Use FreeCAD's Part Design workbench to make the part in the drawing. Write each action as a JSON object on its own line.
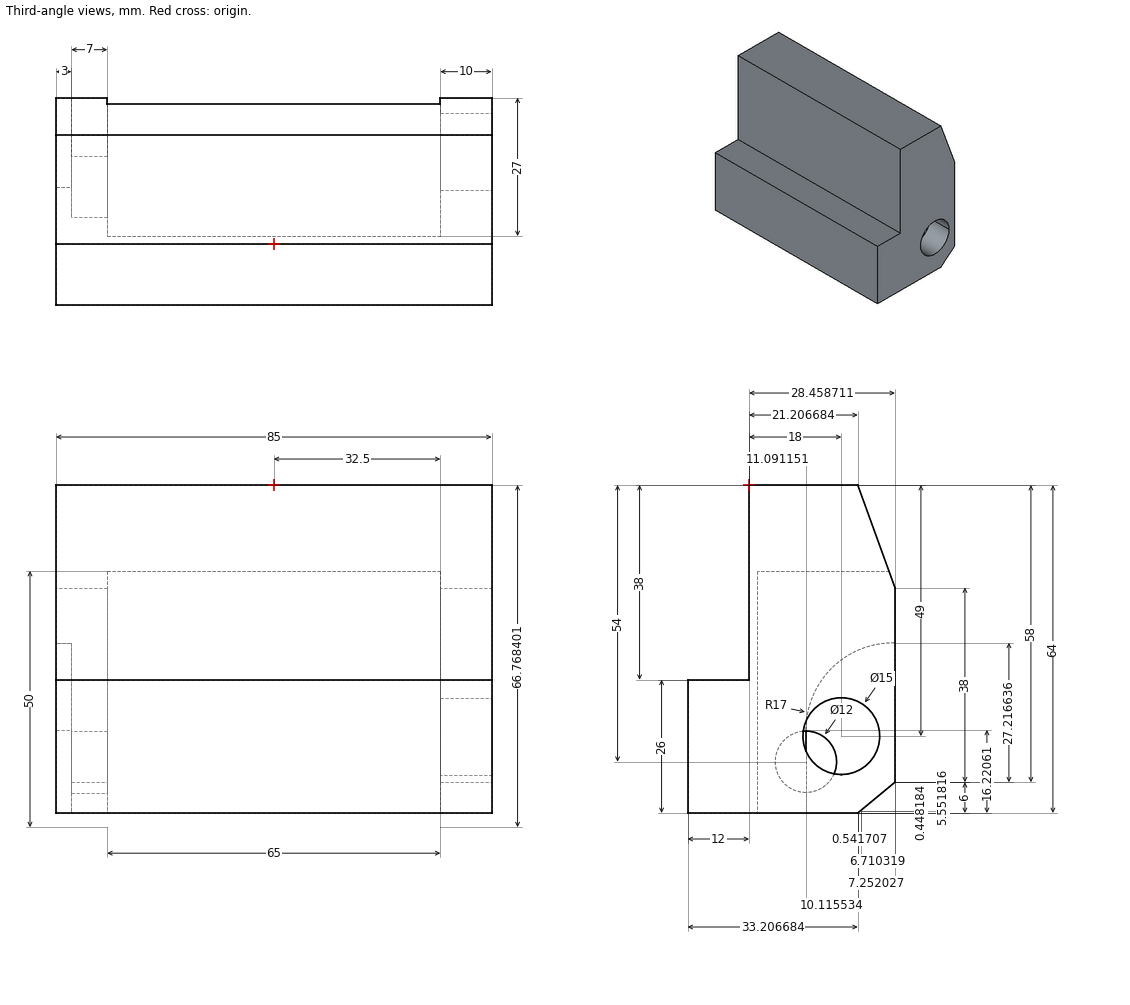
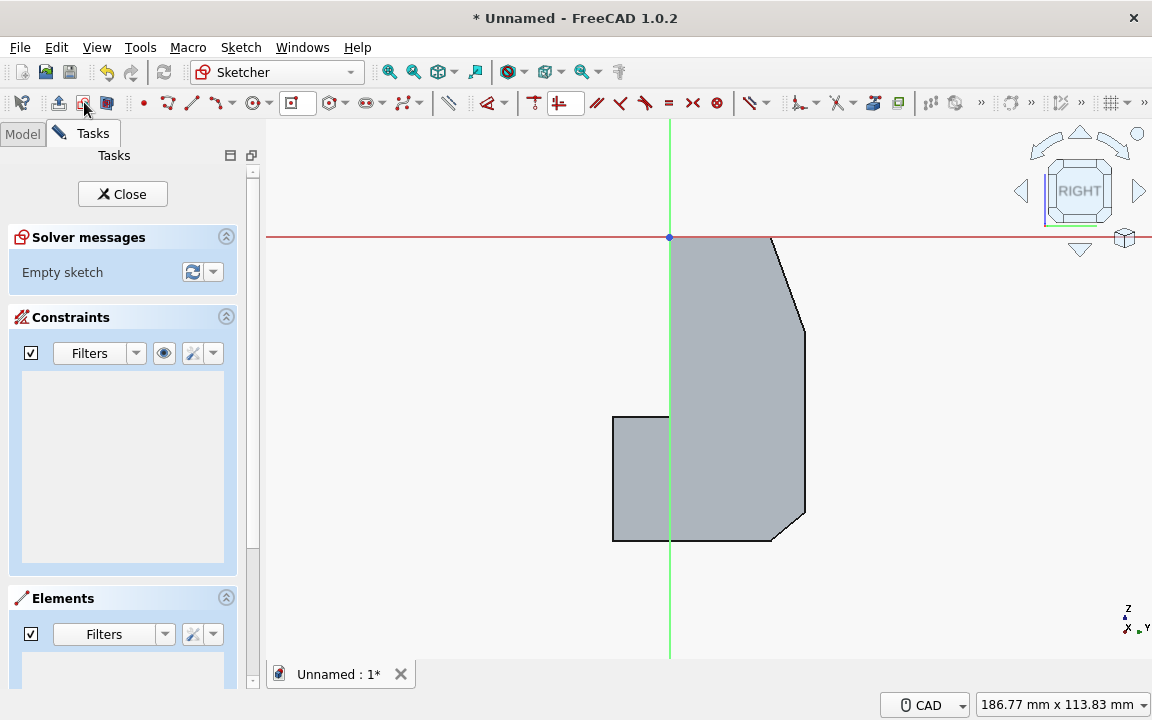
{"action": "scroll", "coordinate": [784, 490], "scroll_direction": "up", "scroll_amount": 8}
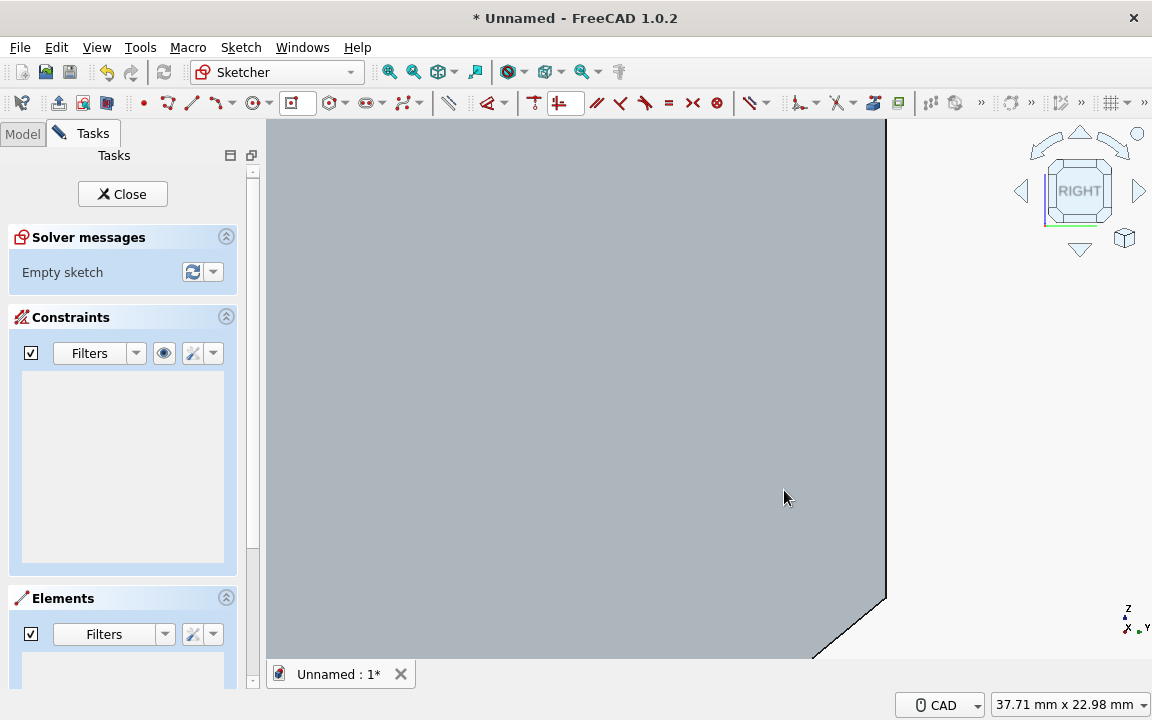
{"action": "left_click", "coordinate": [254, 104]}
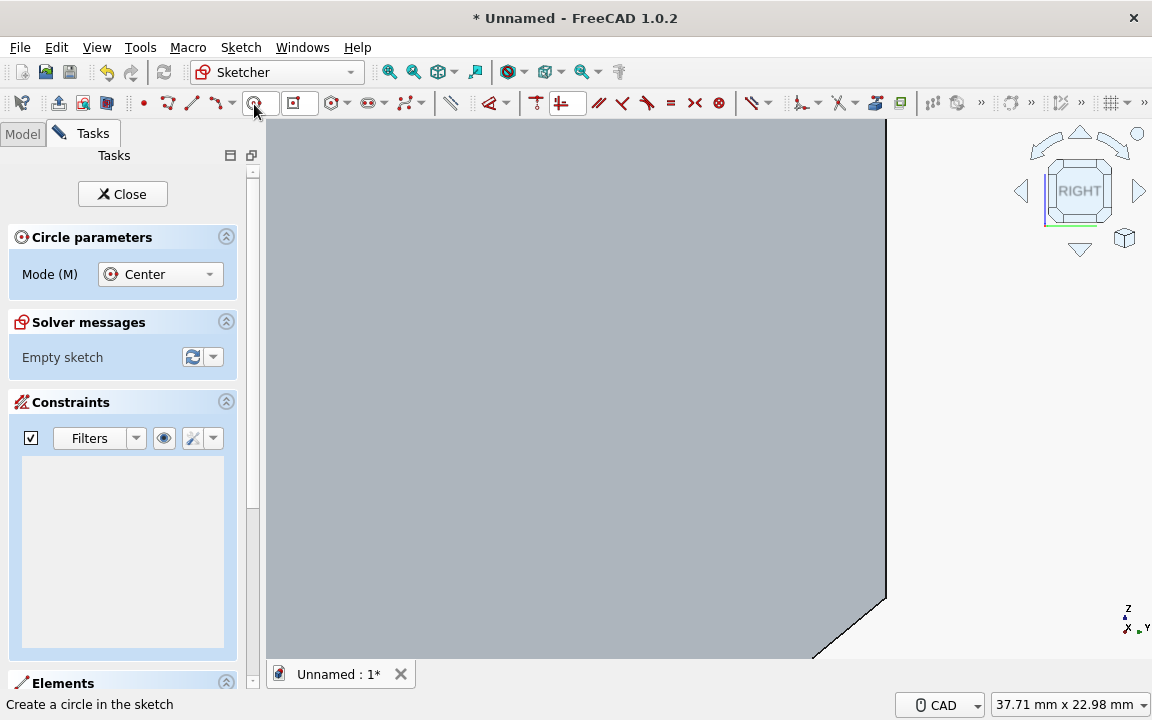
{"action": "left_click", "coordinate": [640, 386]}
{"action": "left_click", "coordinate": [764, 262]}
{"action": "key", "text": "Escape"}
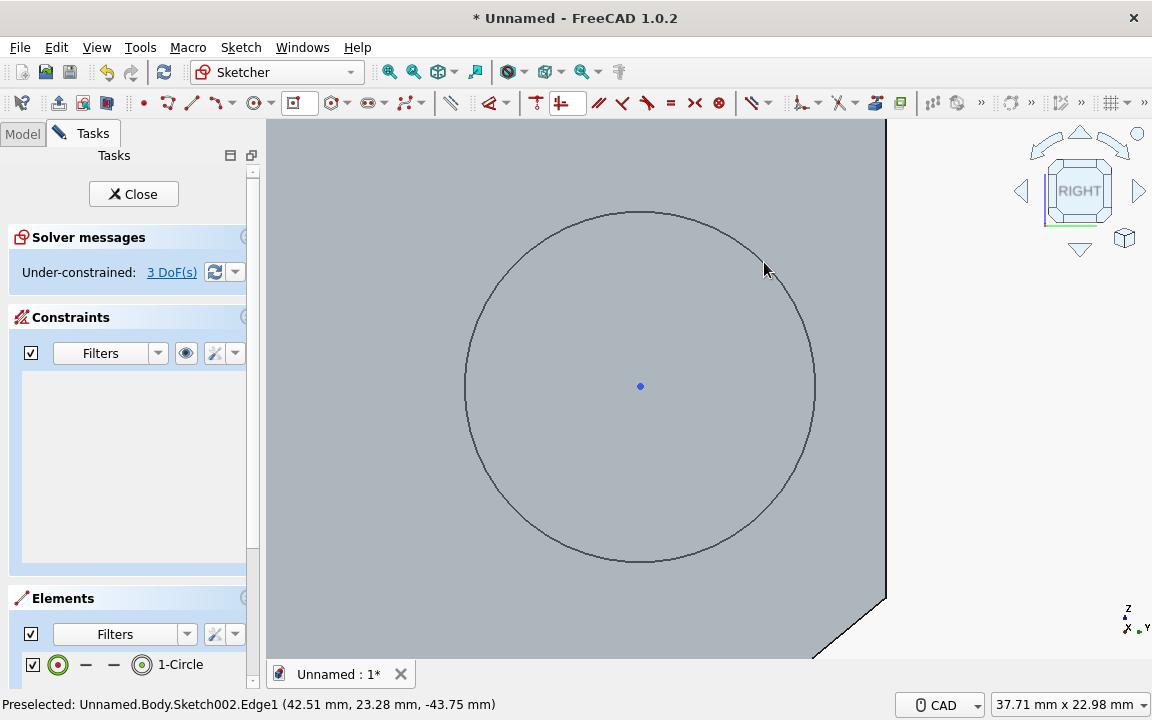
{"action": "left_click", "coordinate": [490, 104]}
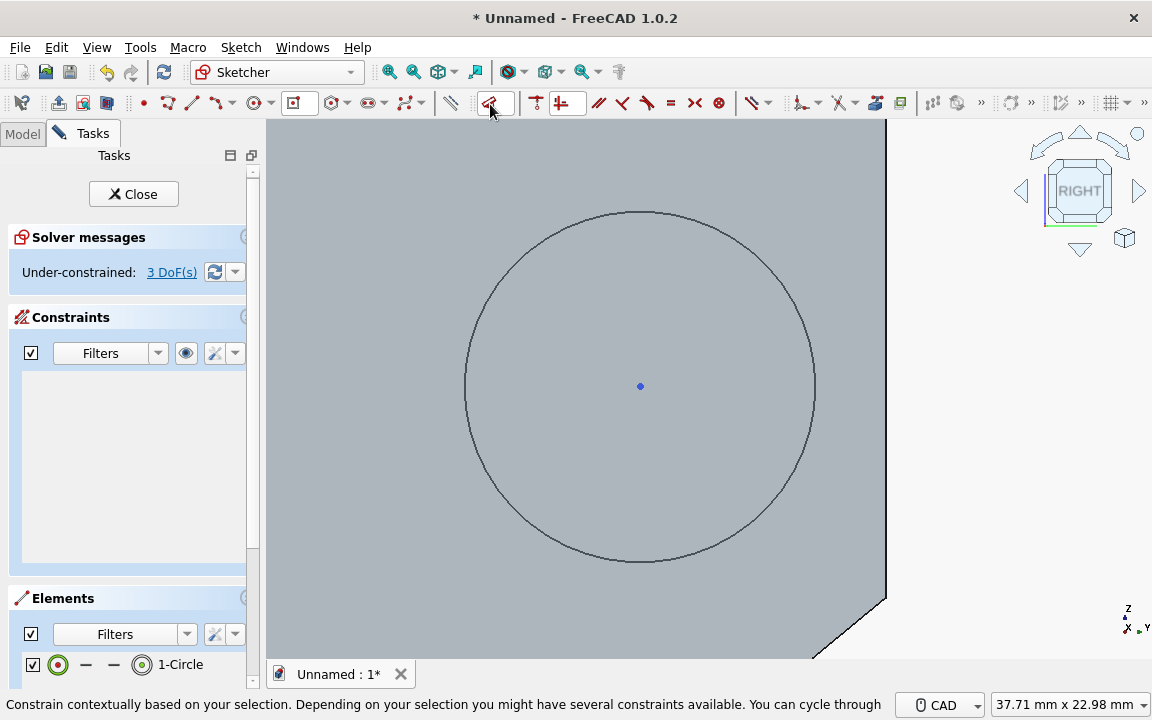
{"action": "left_click", "coordinate": [764, 263]}
{"action": "left_click", "coordinate": [787, 240]}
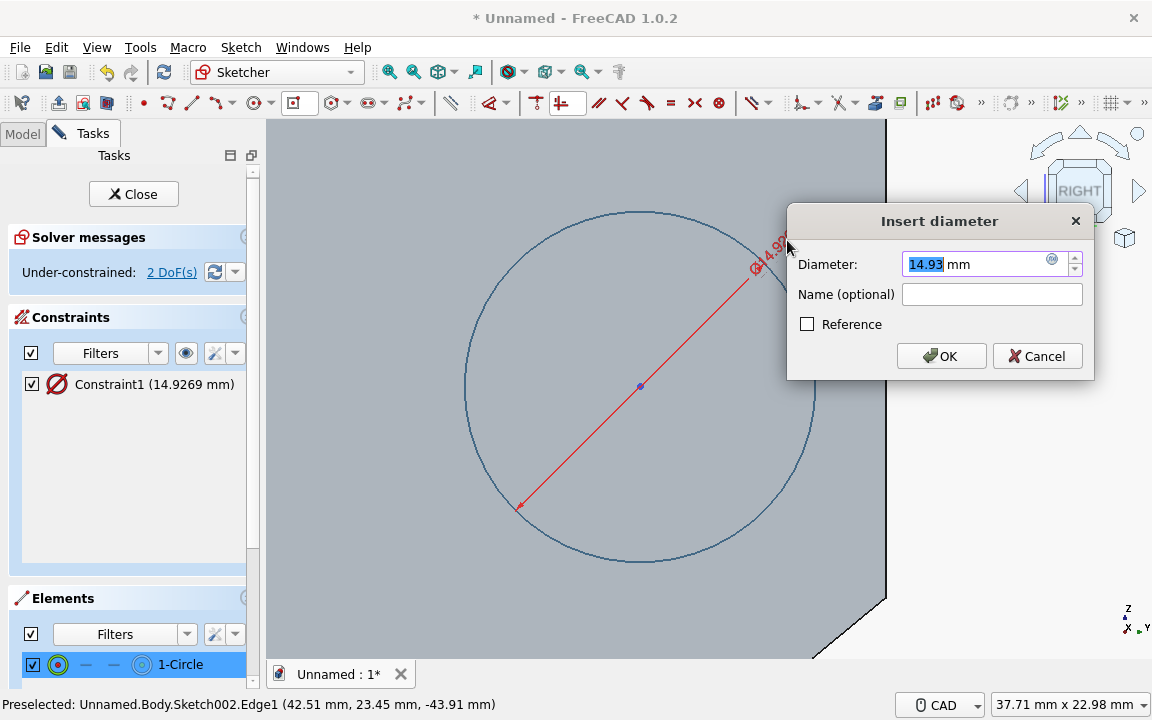
{"action": "type", "text": "15"}
{"action": "key", "text": "Return"}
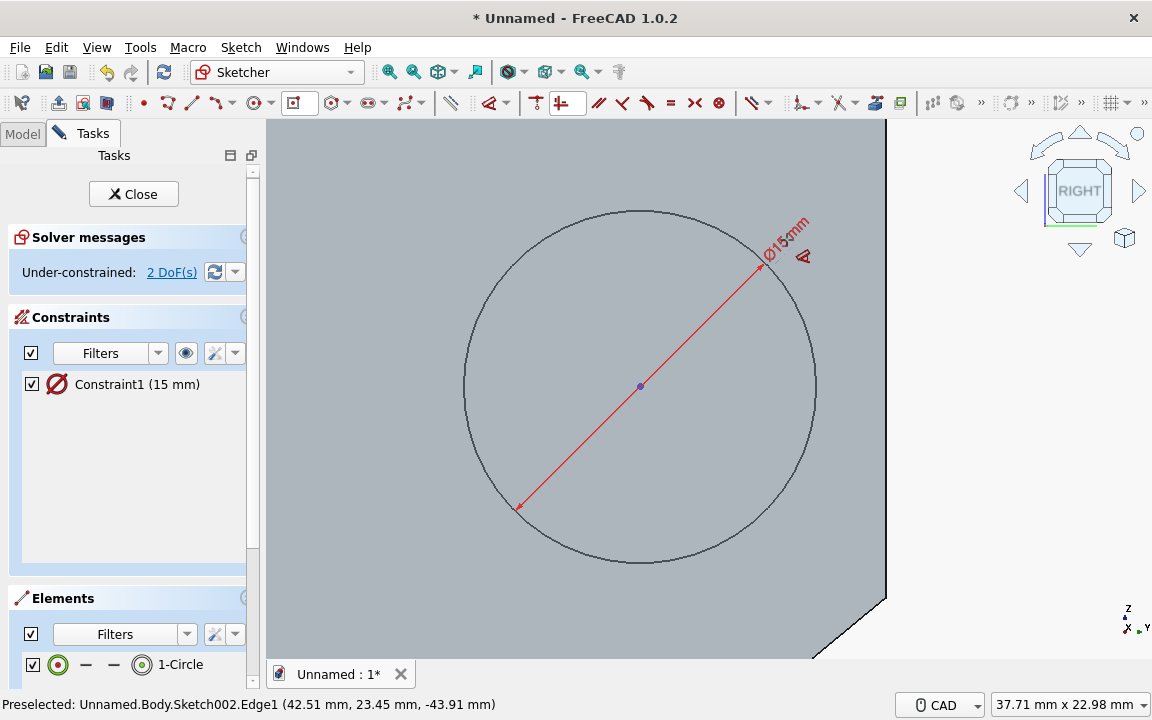
{"action": "left_click", "coordinate": [640, 387]}
{"action": "left_click", "coordinate": [387, 421]}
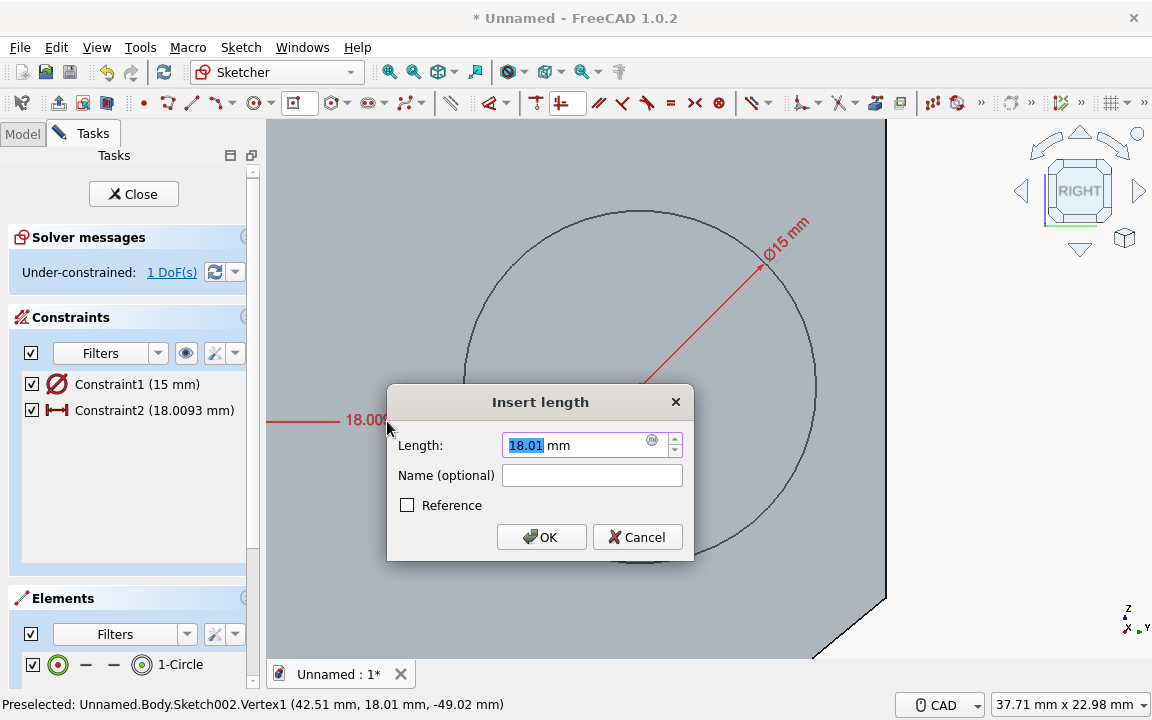
{"action": "type", "text": "18"}
{"action": "key", "text": "Return"}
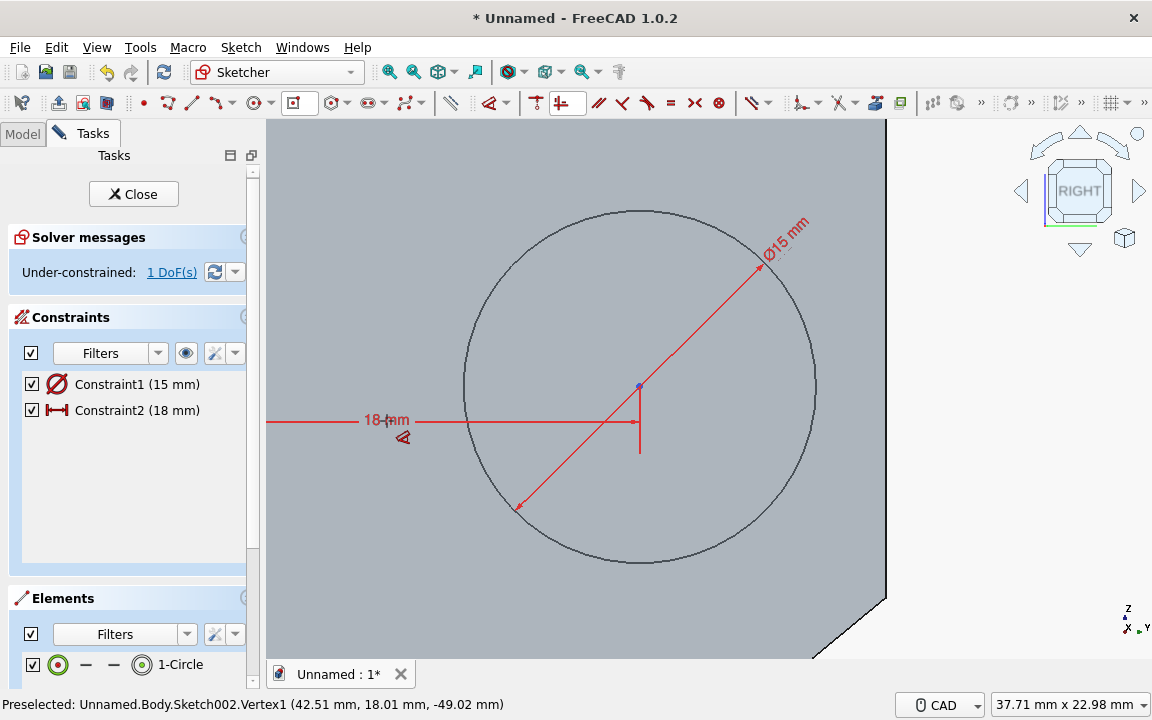
{"action": "left_click", "coordinate": [640, 387]}
{"action": "left_click", "coordinate": [674, 267]}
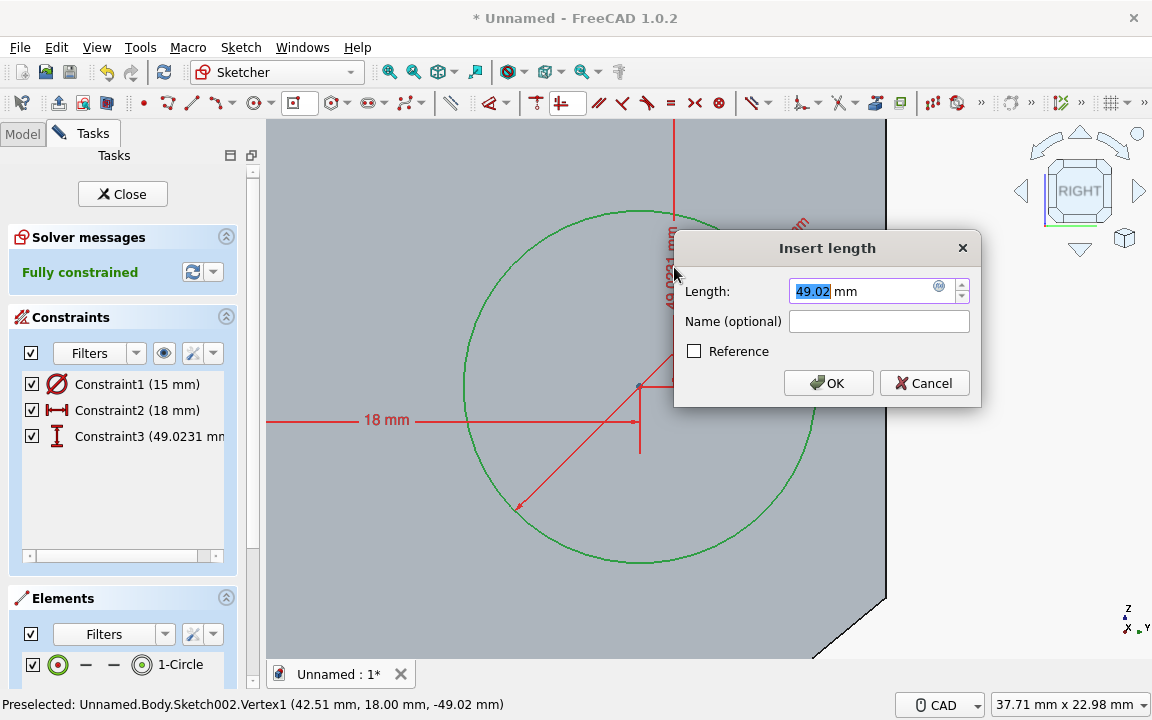
{"action": "type", "text": "49"}
{"action": "key", "text": "Return"}
{"action": "key", "text": "Escape"}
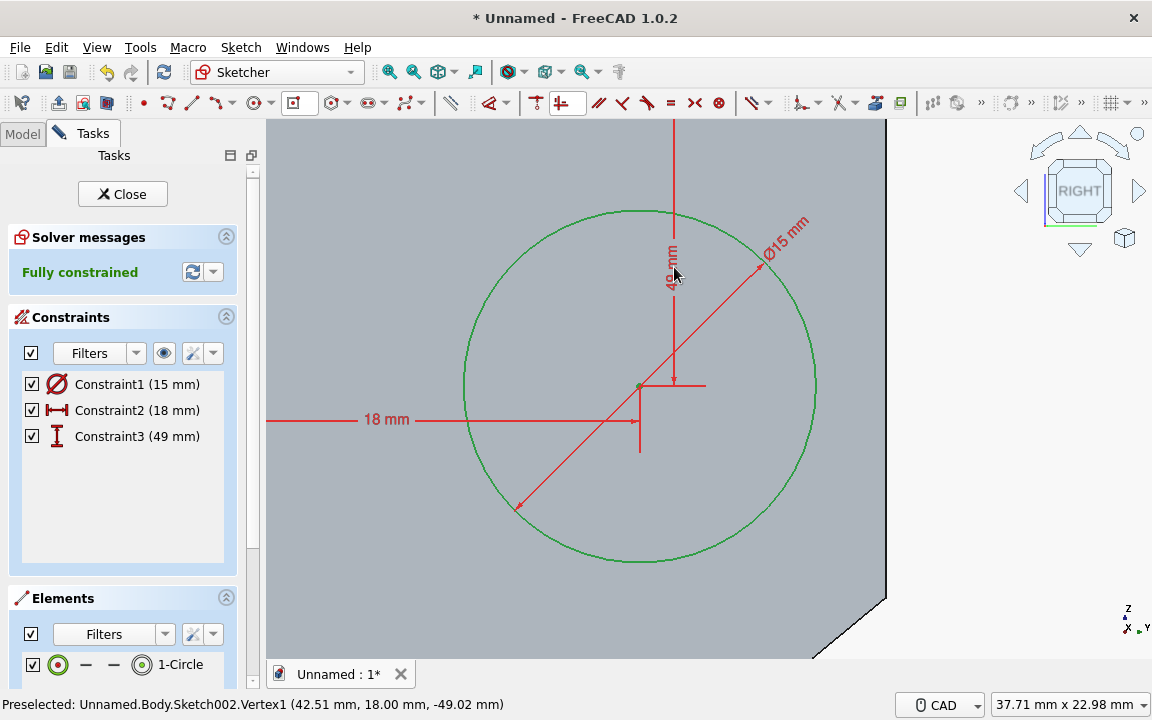
{"action": "left_click", "coordinate": [123, 194]}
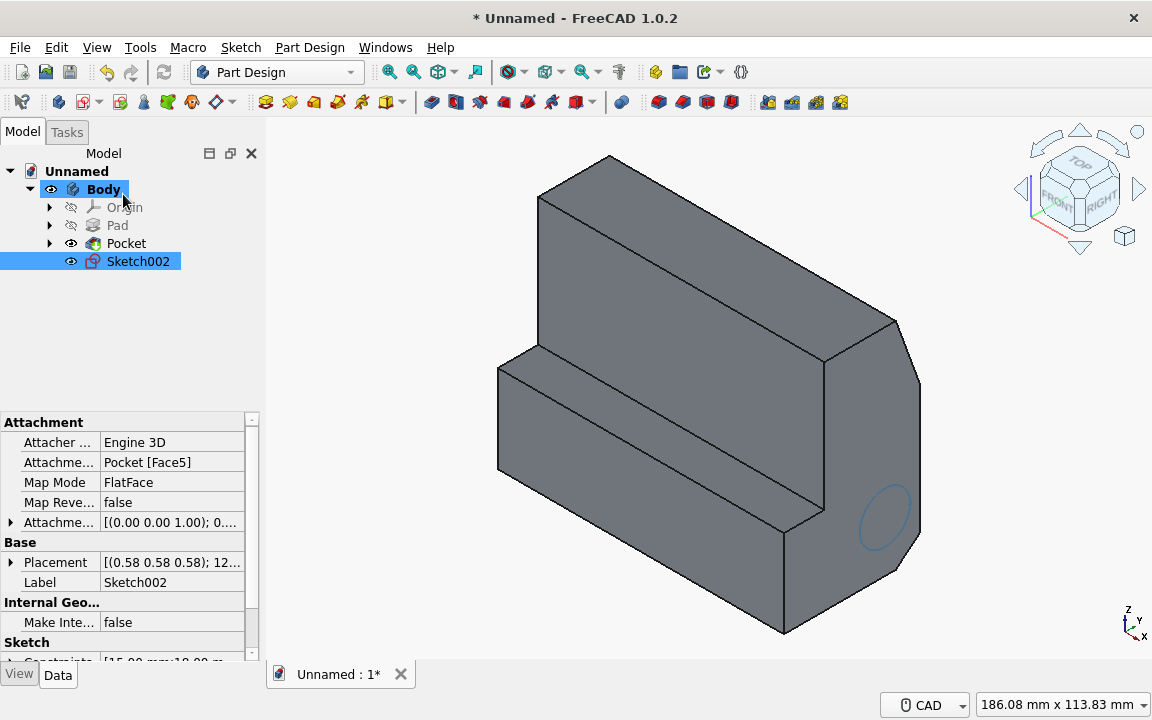
{"action": "left_click", "coordinate": [432, 102]}